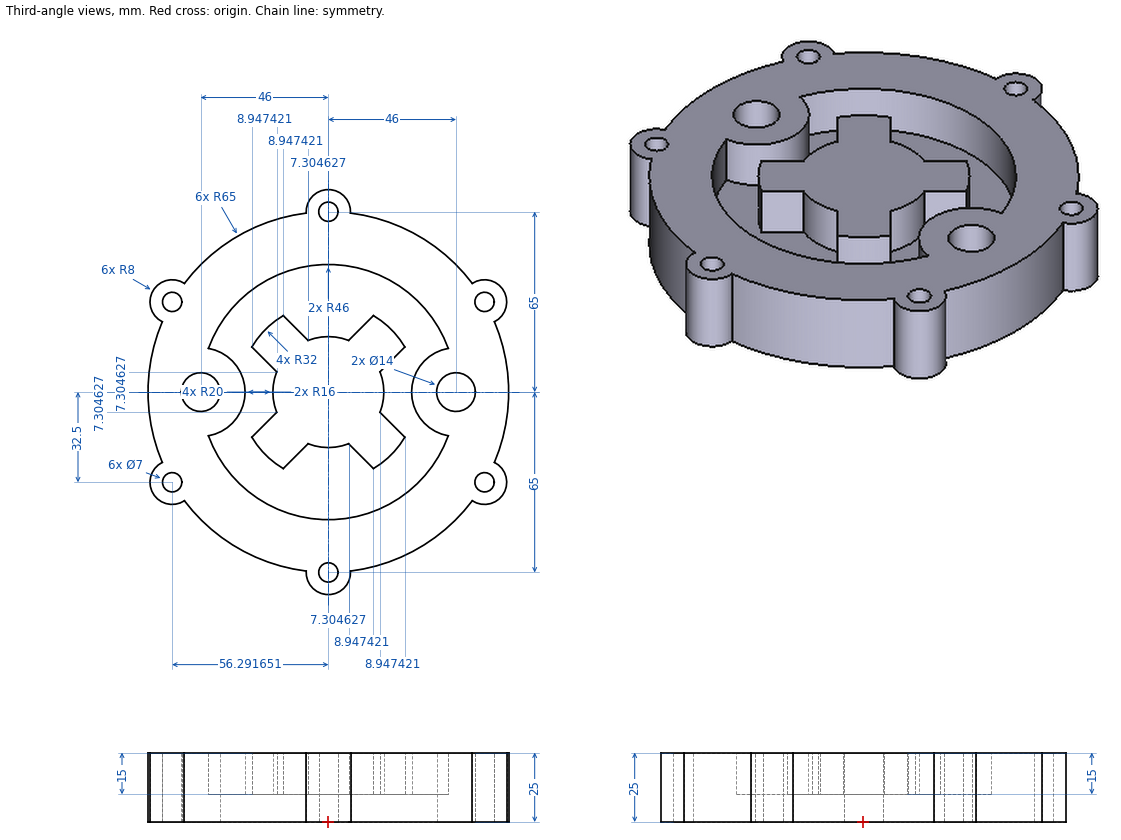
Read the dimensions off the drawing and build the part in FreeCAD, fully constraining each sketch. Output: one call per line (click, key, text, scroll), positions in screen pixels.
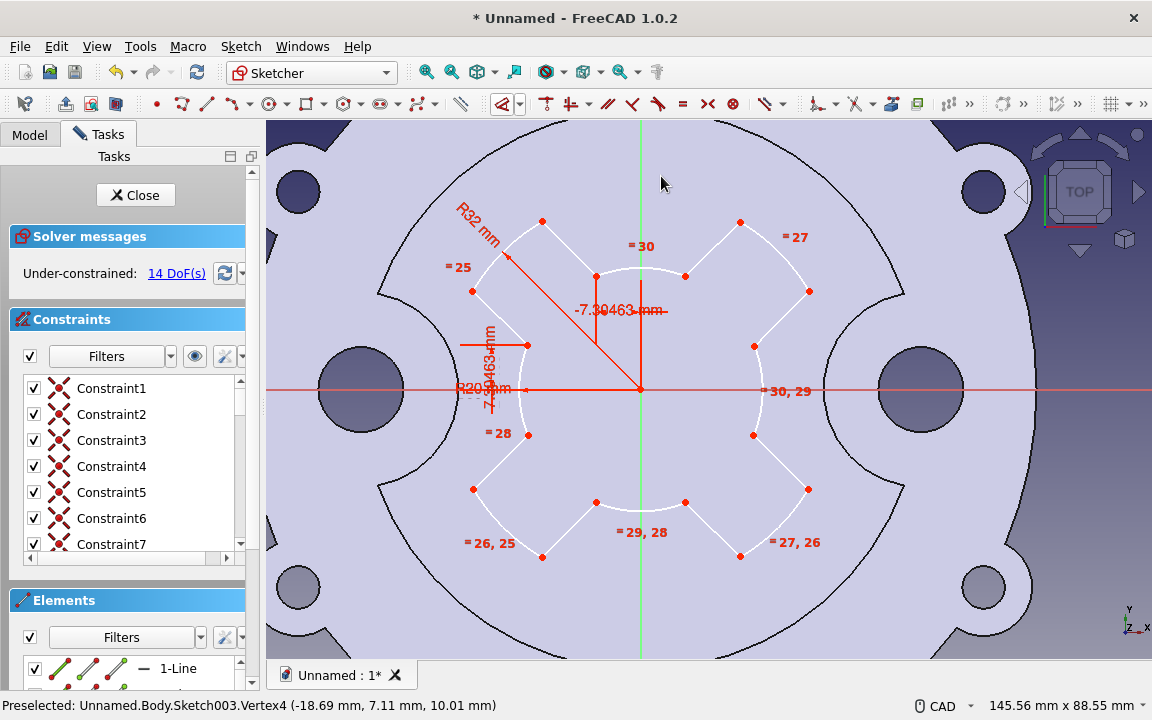
click(528, 435)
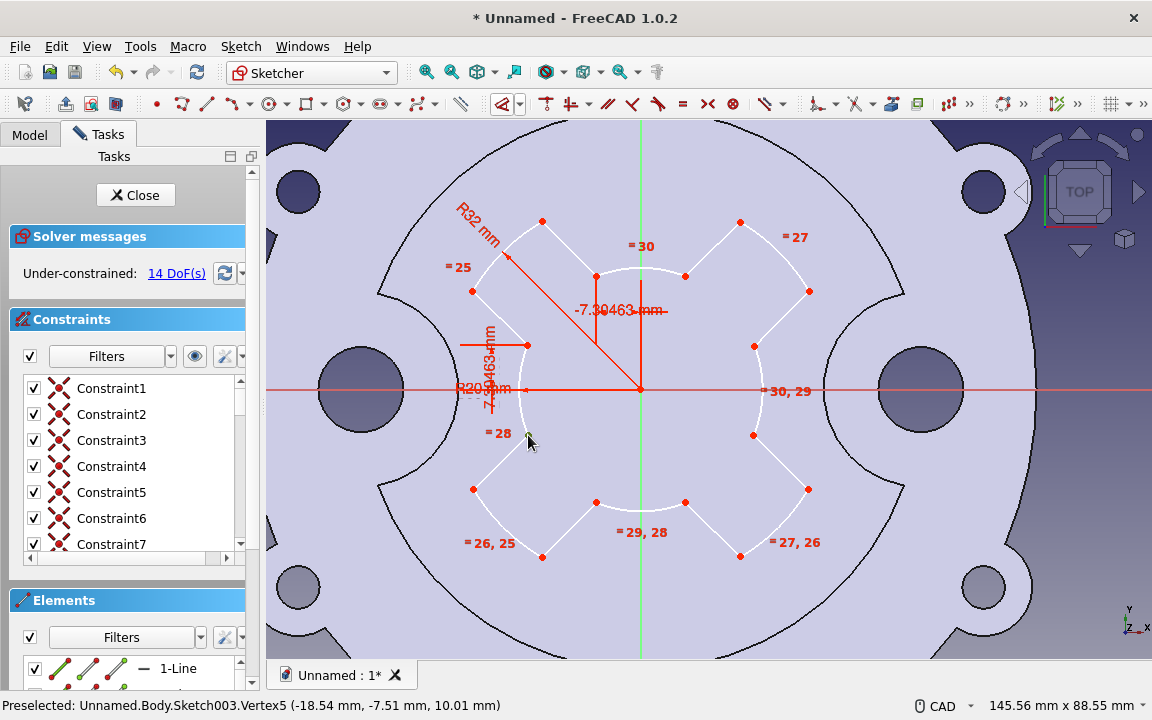
key(i)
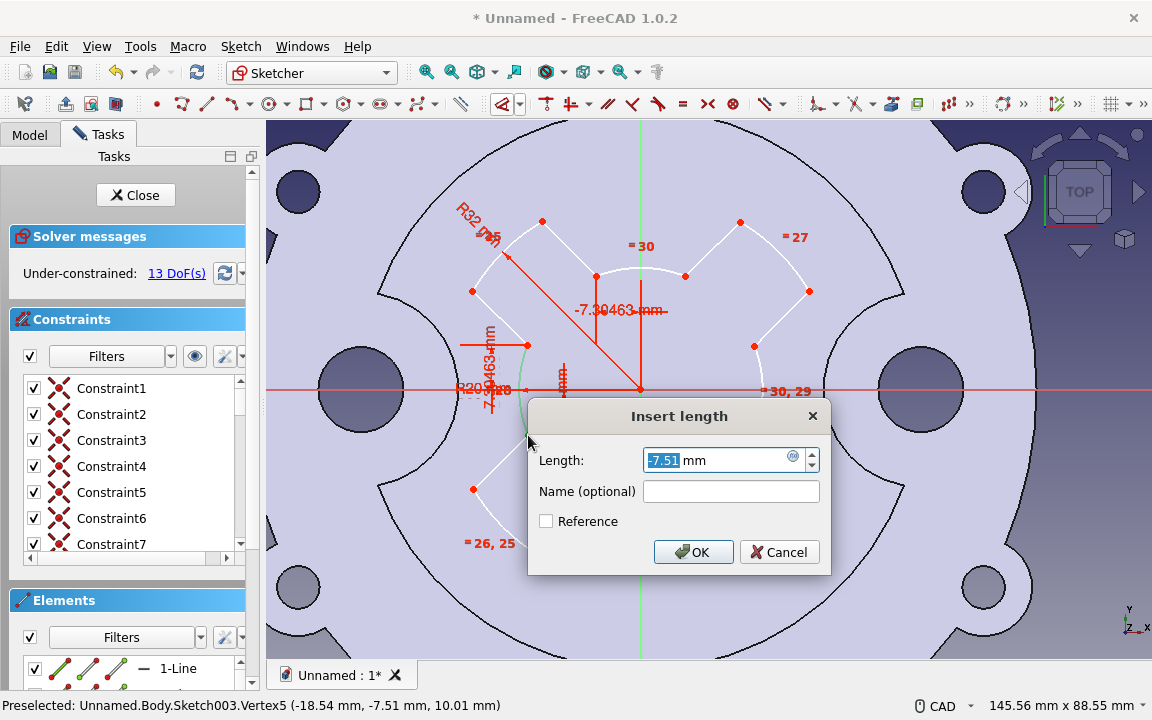
text(-7.304627)
key(Return)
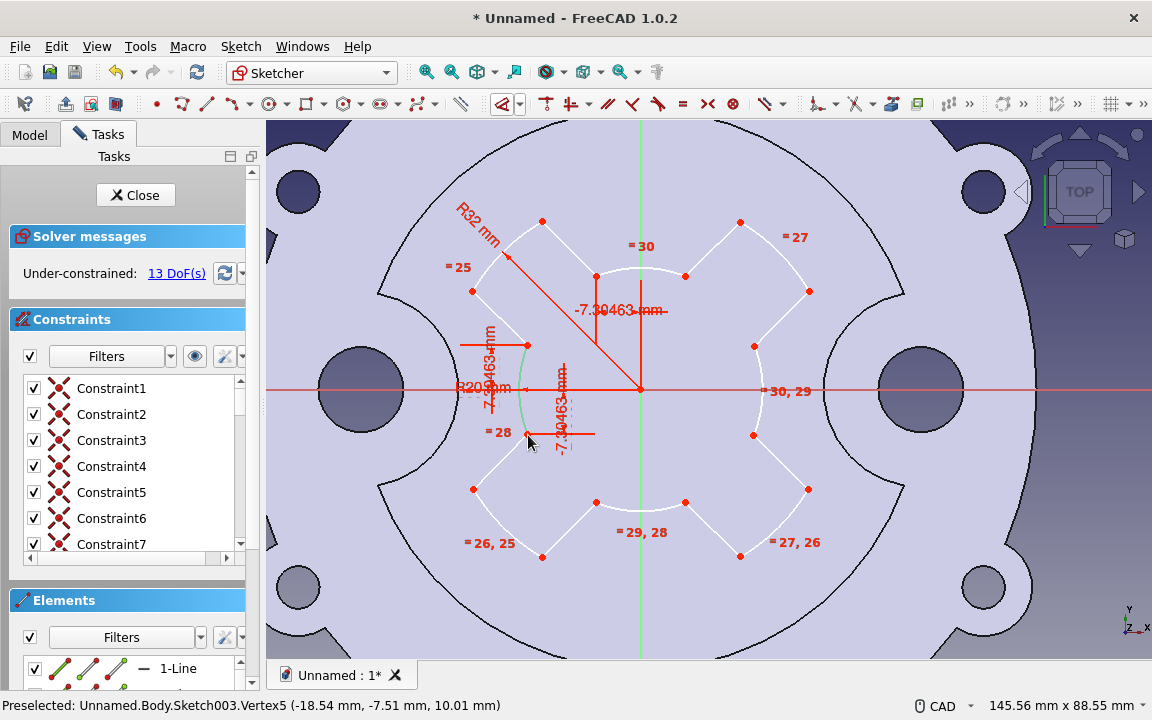
click(596, 503)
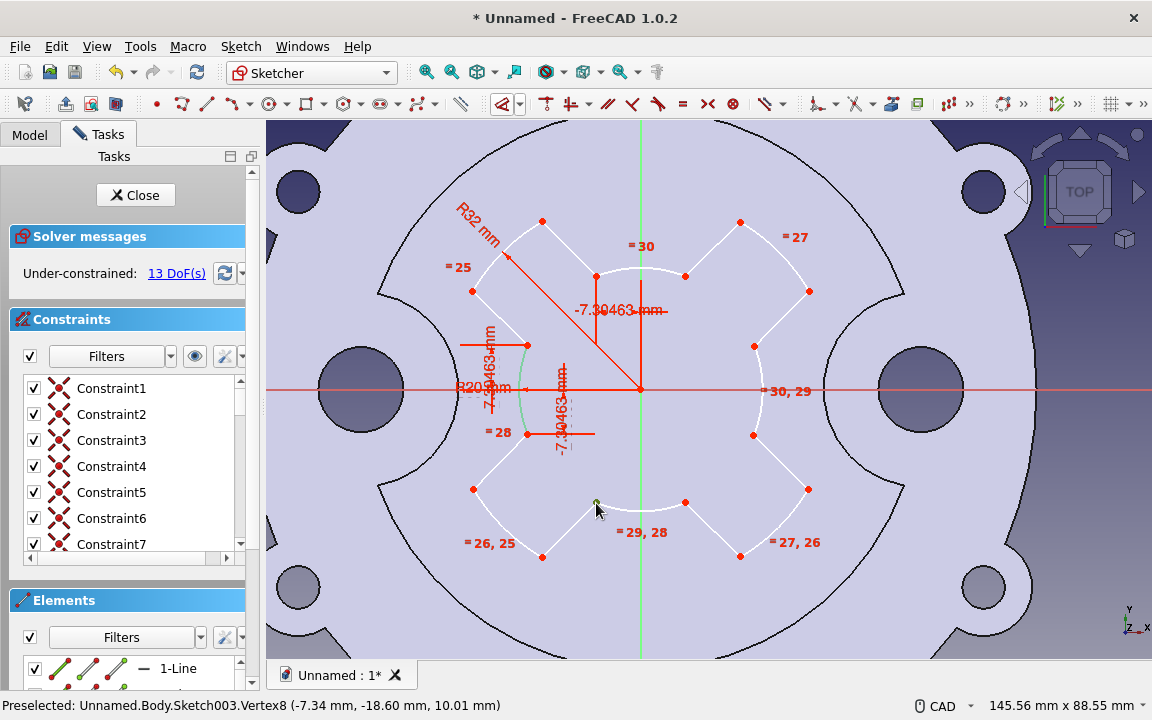
click(520, 104)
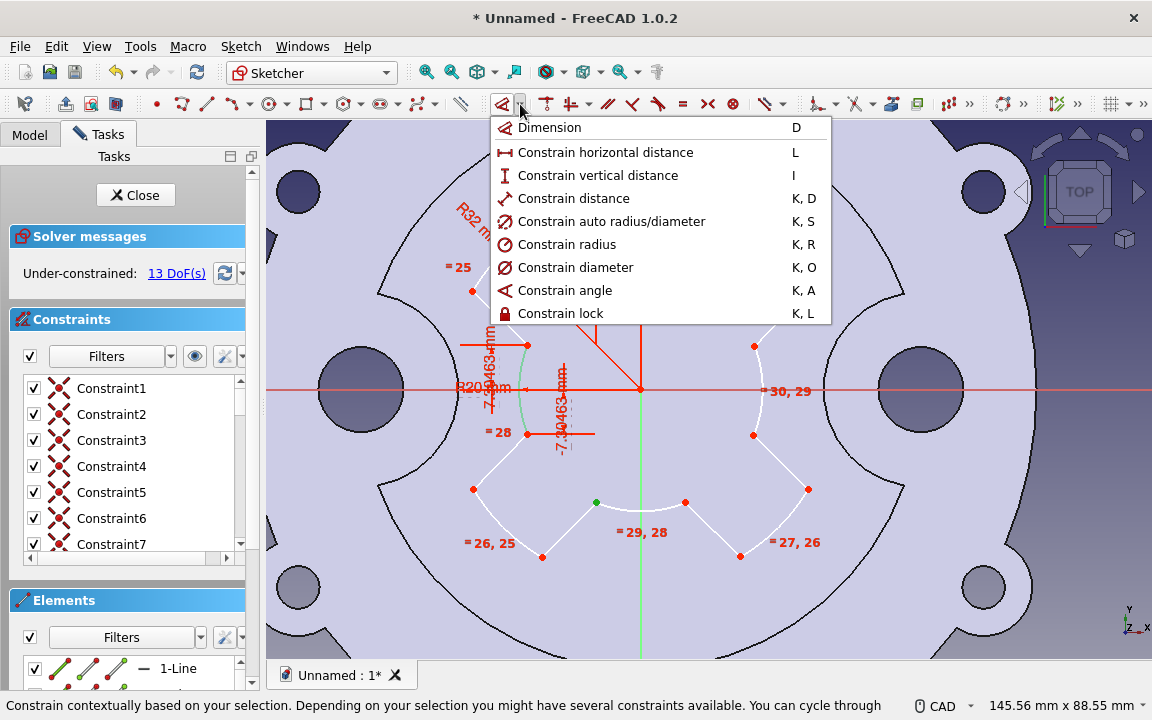
click(661, 152)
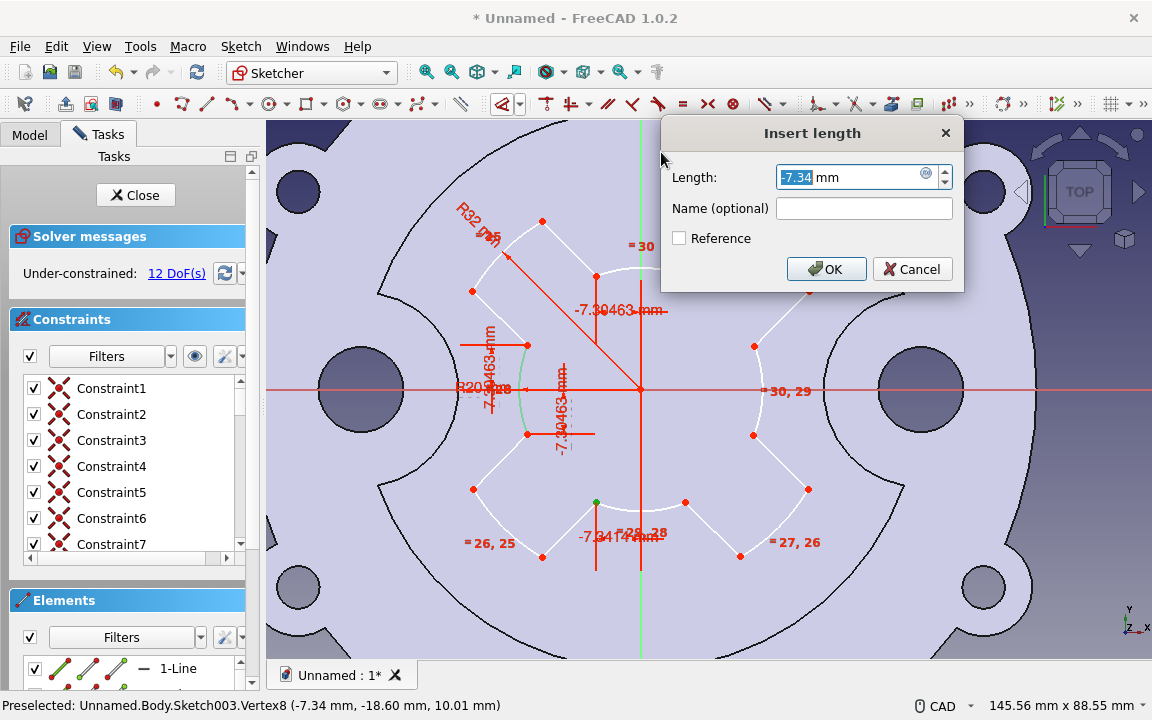
text(-7.304627)
key(Return)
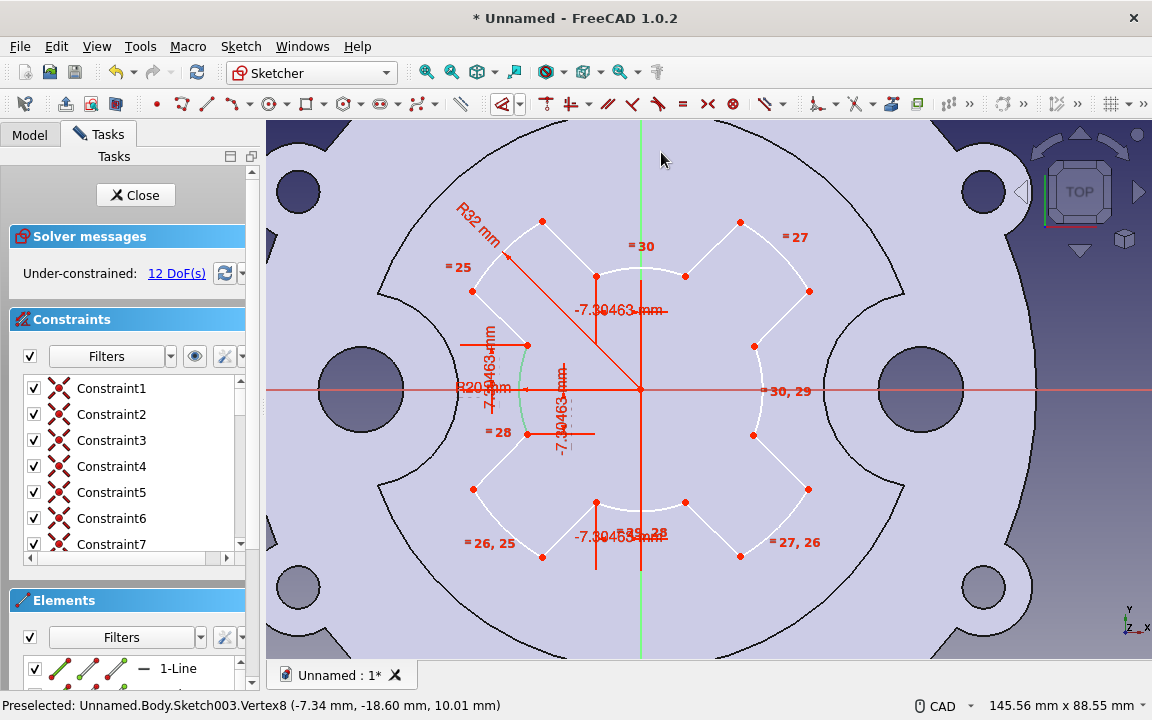
click(685, 503)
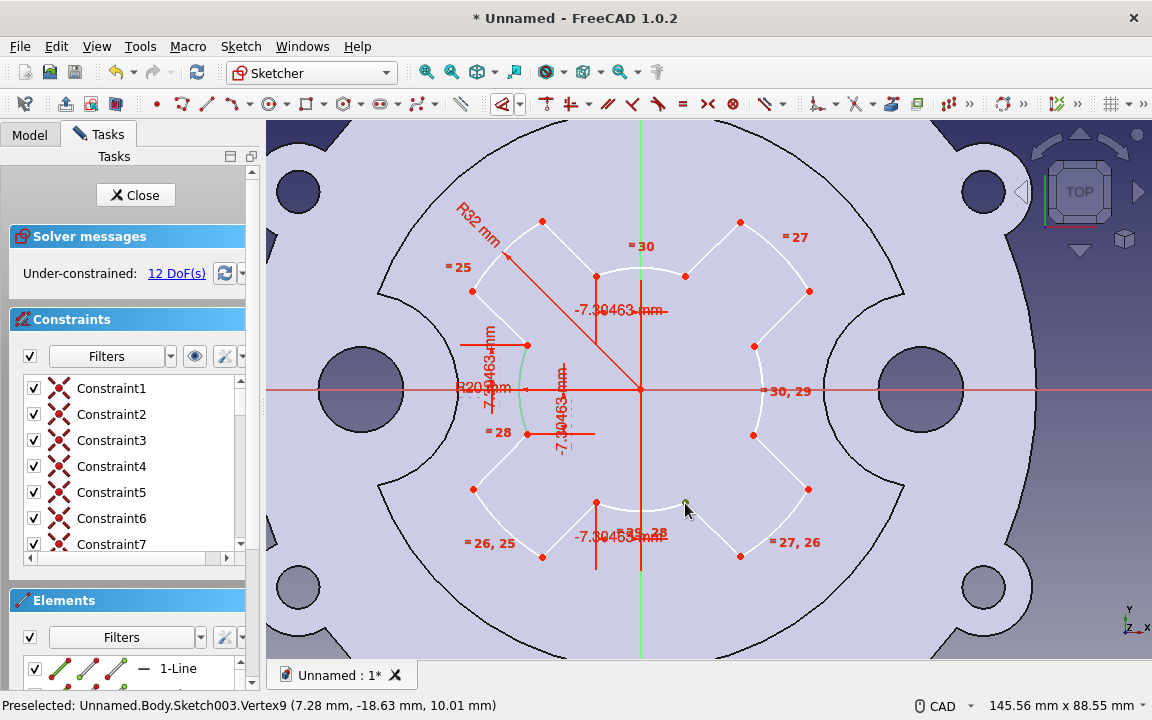
click(520, 104)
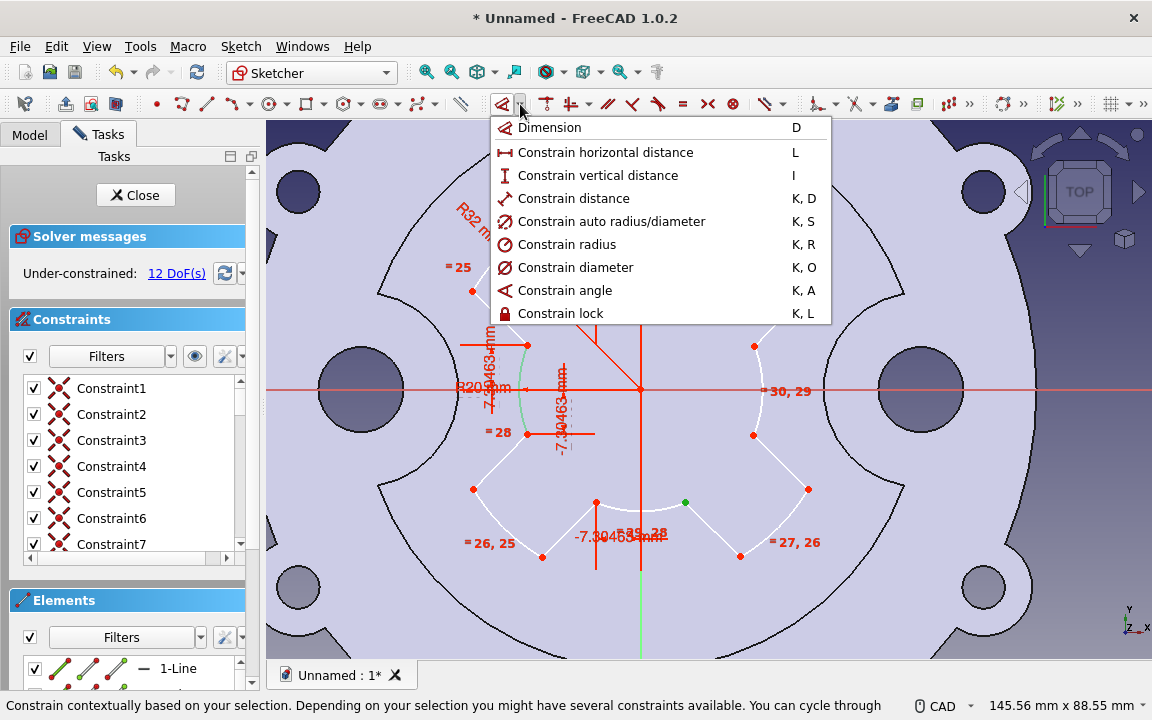
click(661, 152)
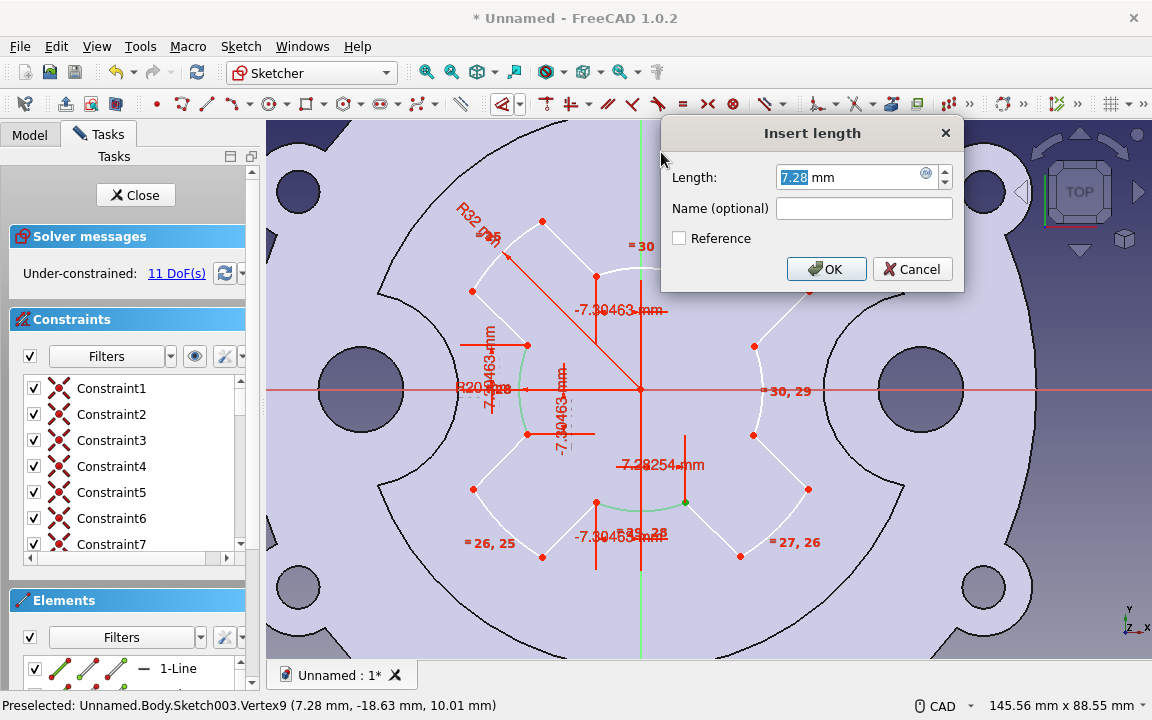
text(7.304627)
key(Return)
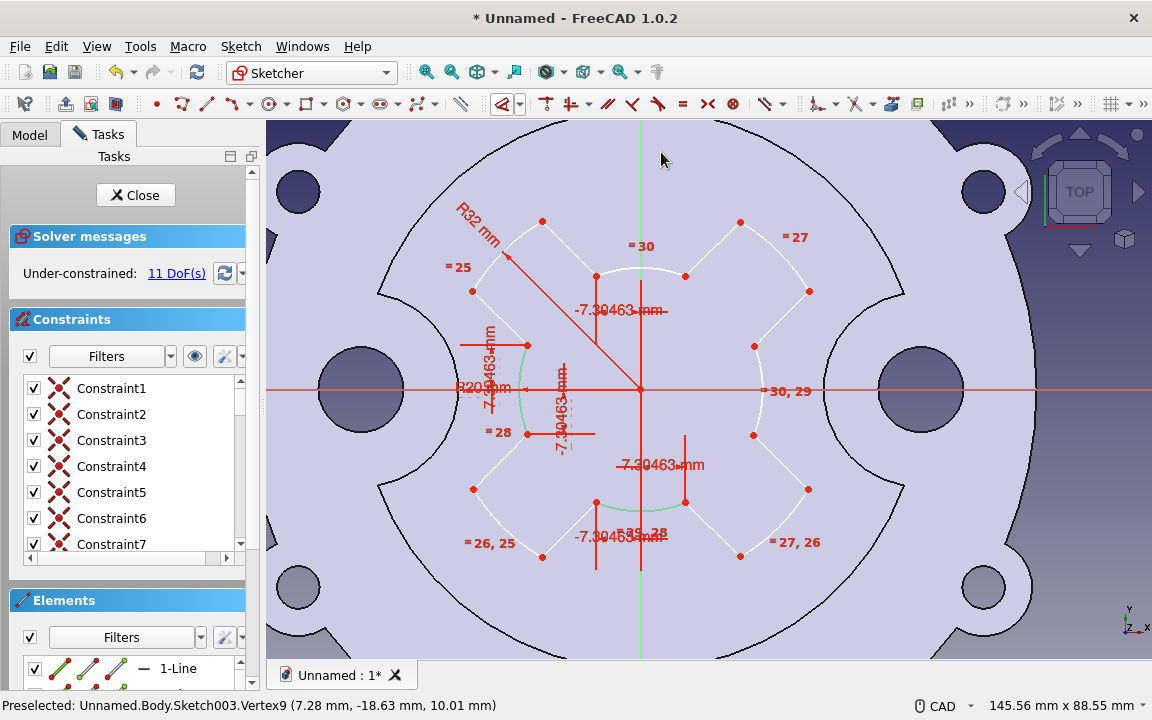
click(754, 435)